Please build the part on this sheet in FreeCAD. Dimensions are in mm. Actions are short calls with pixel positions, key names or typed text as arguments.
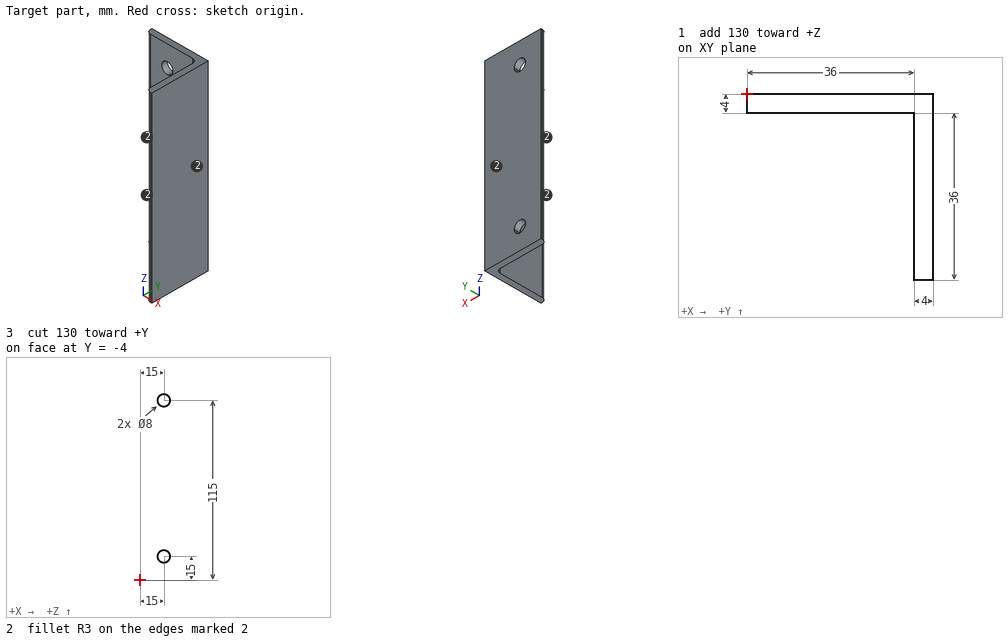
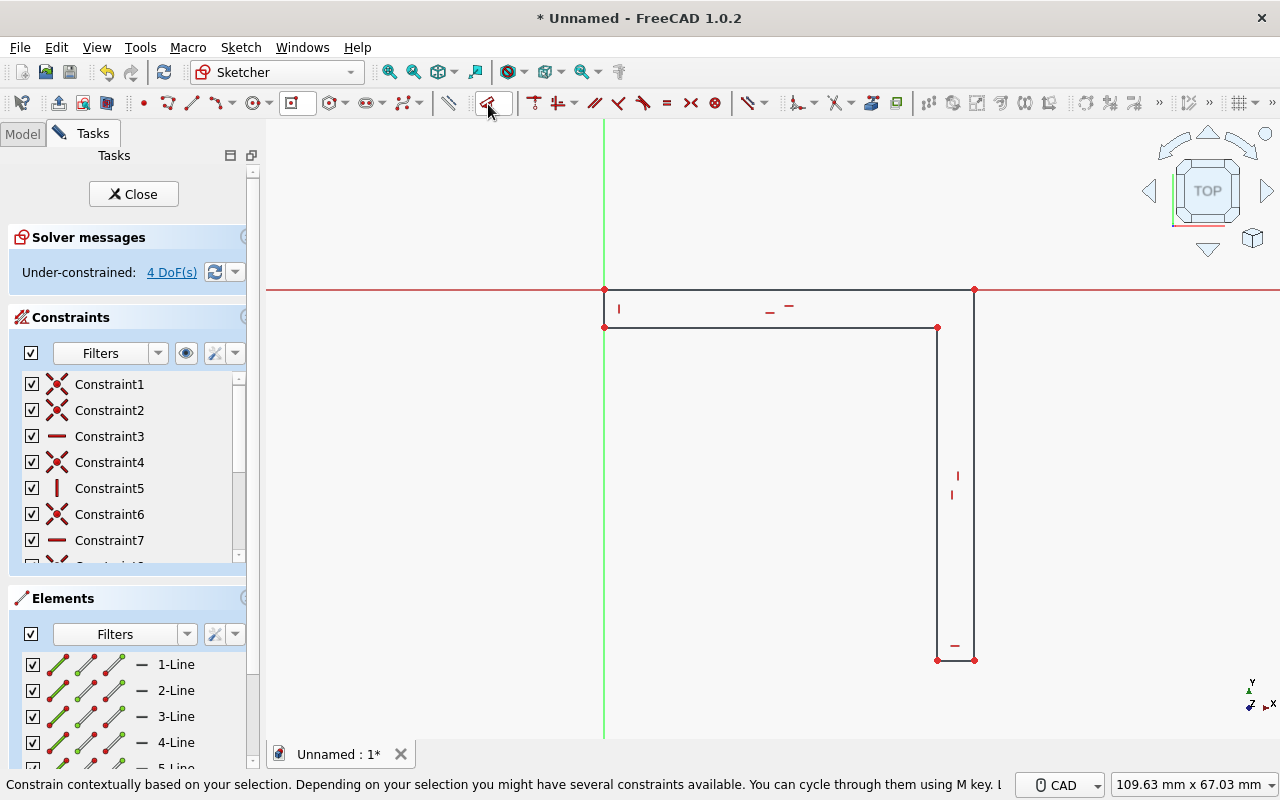
click(604, 301)
click(570, 309)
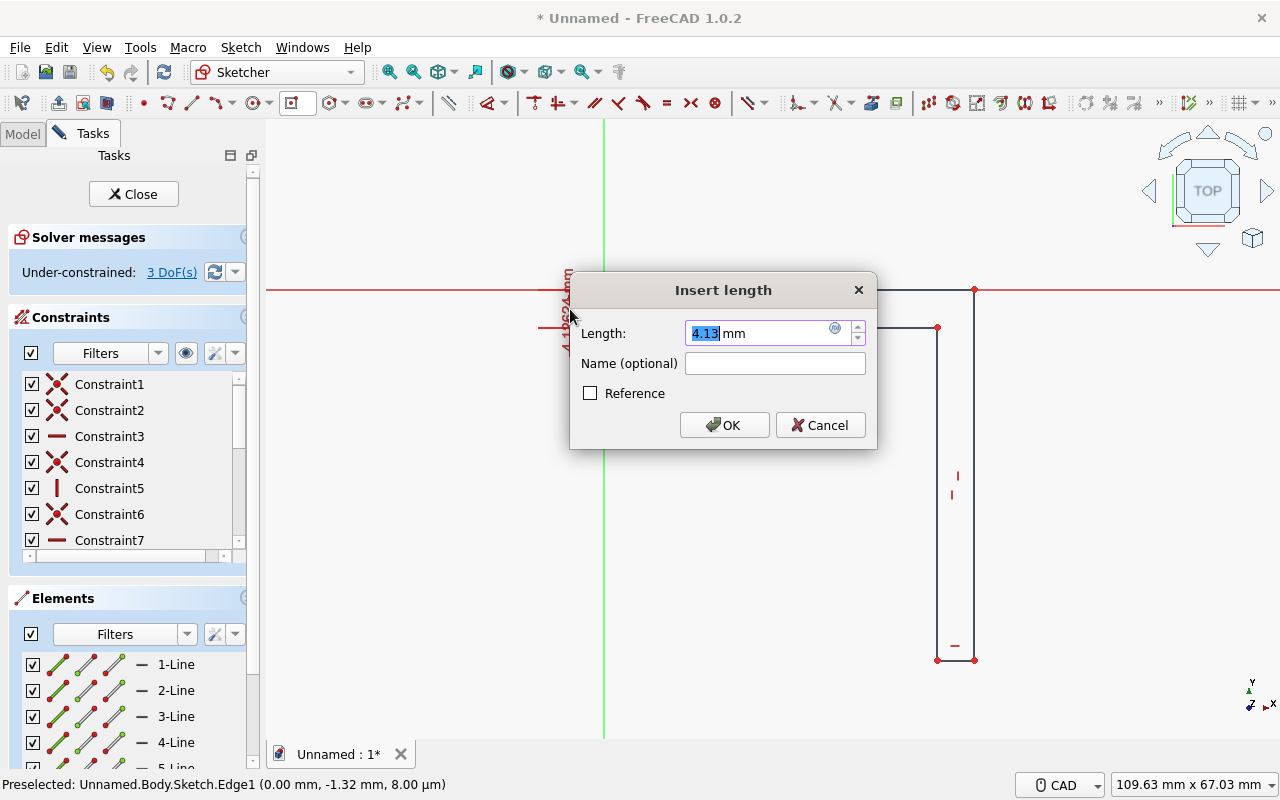
text(4)
key(Return)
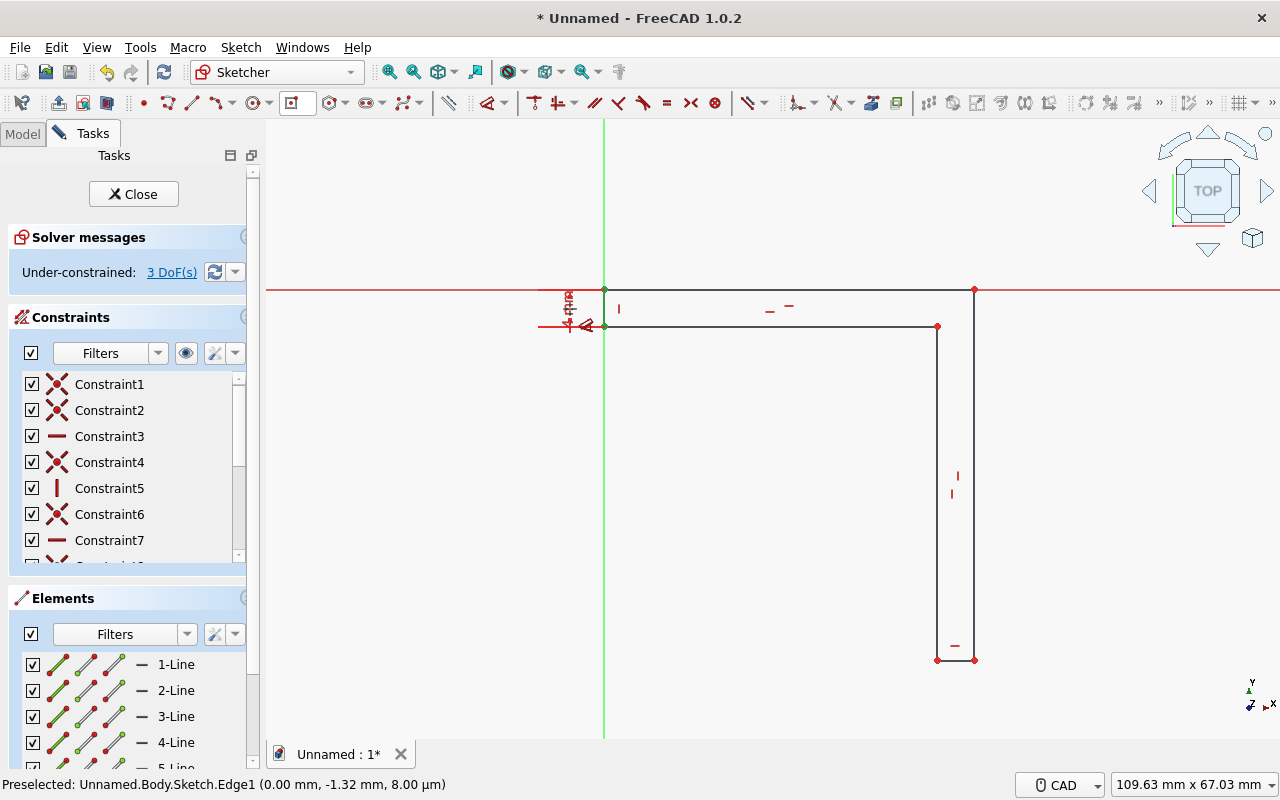
scroll(948, 661, up, 2)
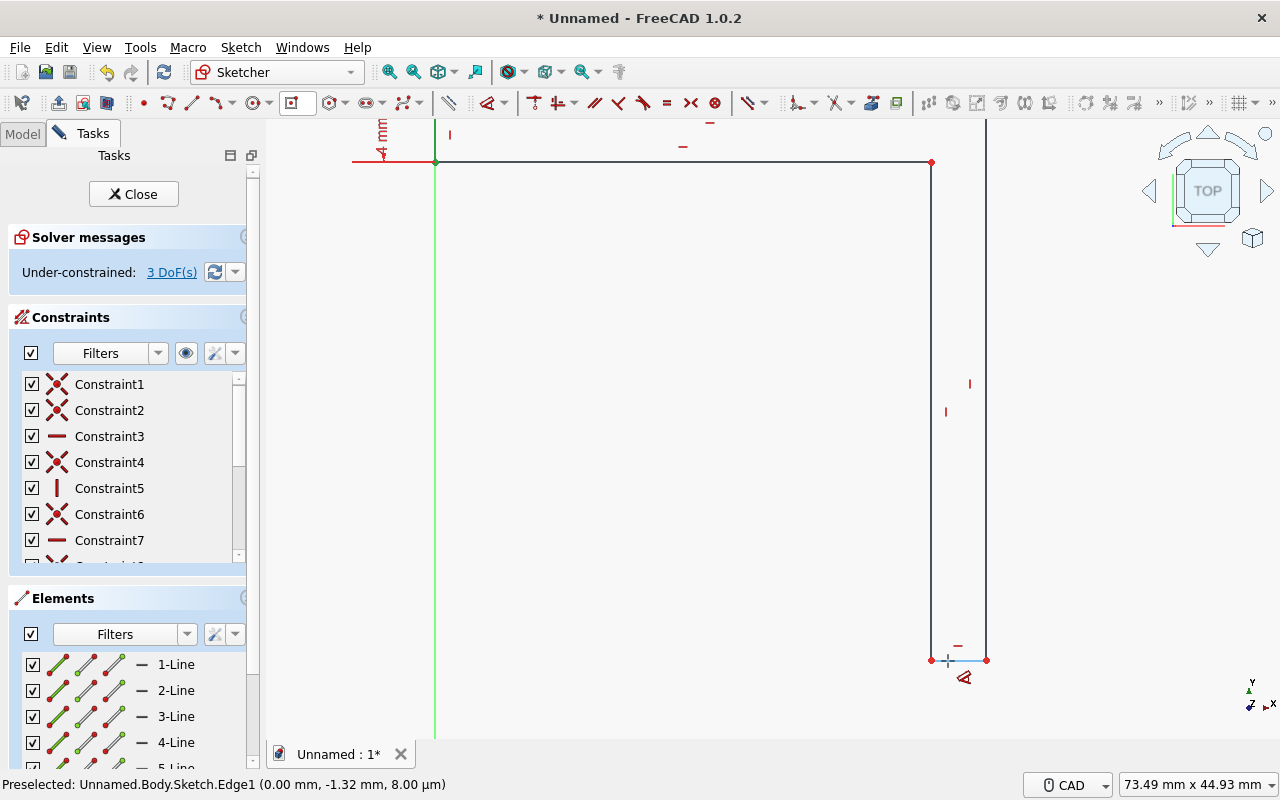
click(948, 661)
click(959, 695)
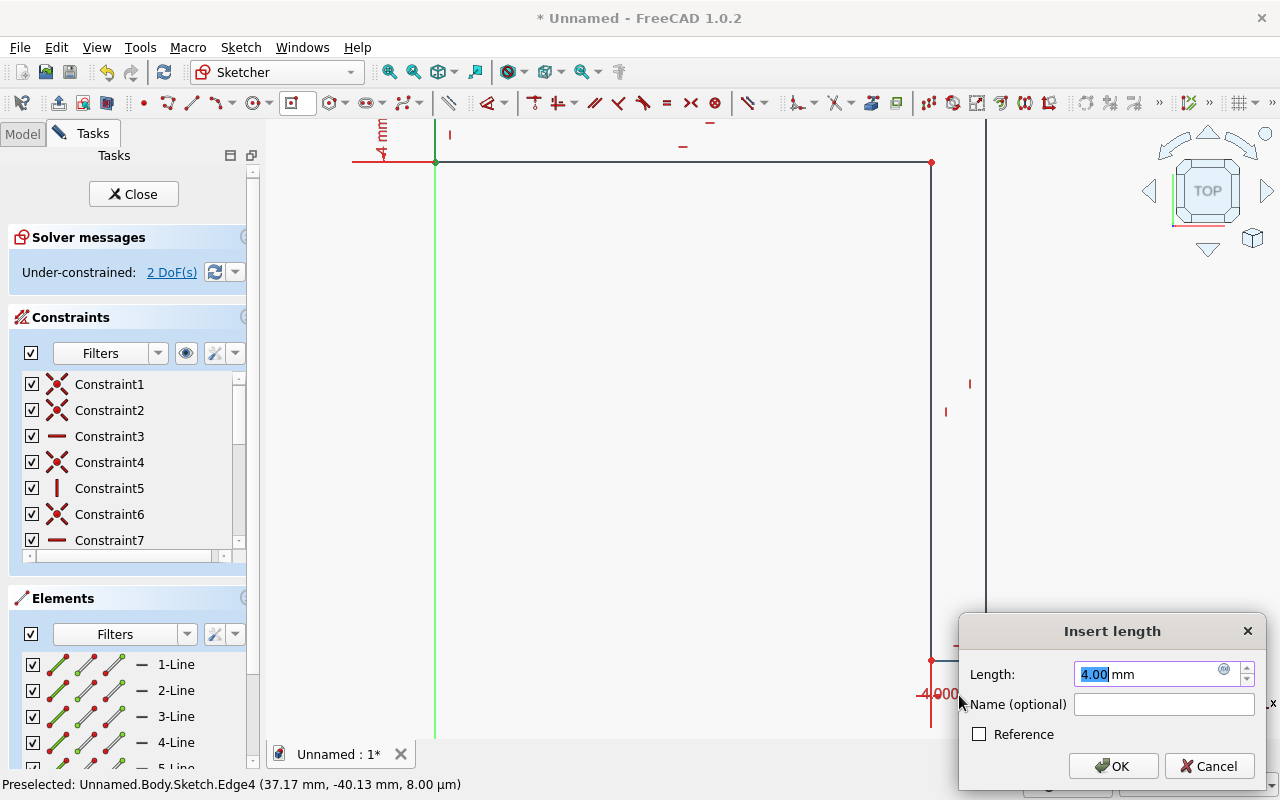
text(4)
key(Return)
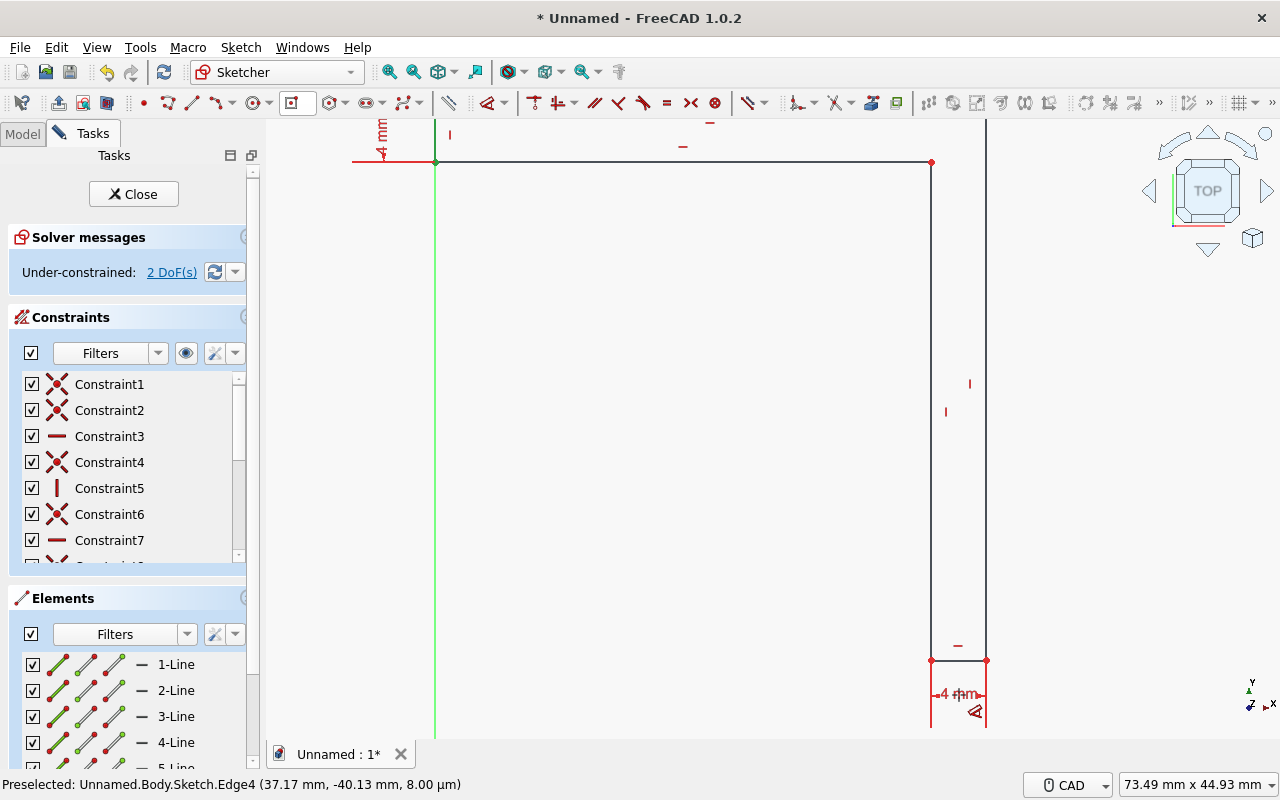
click(584, 162)
click(683, 196)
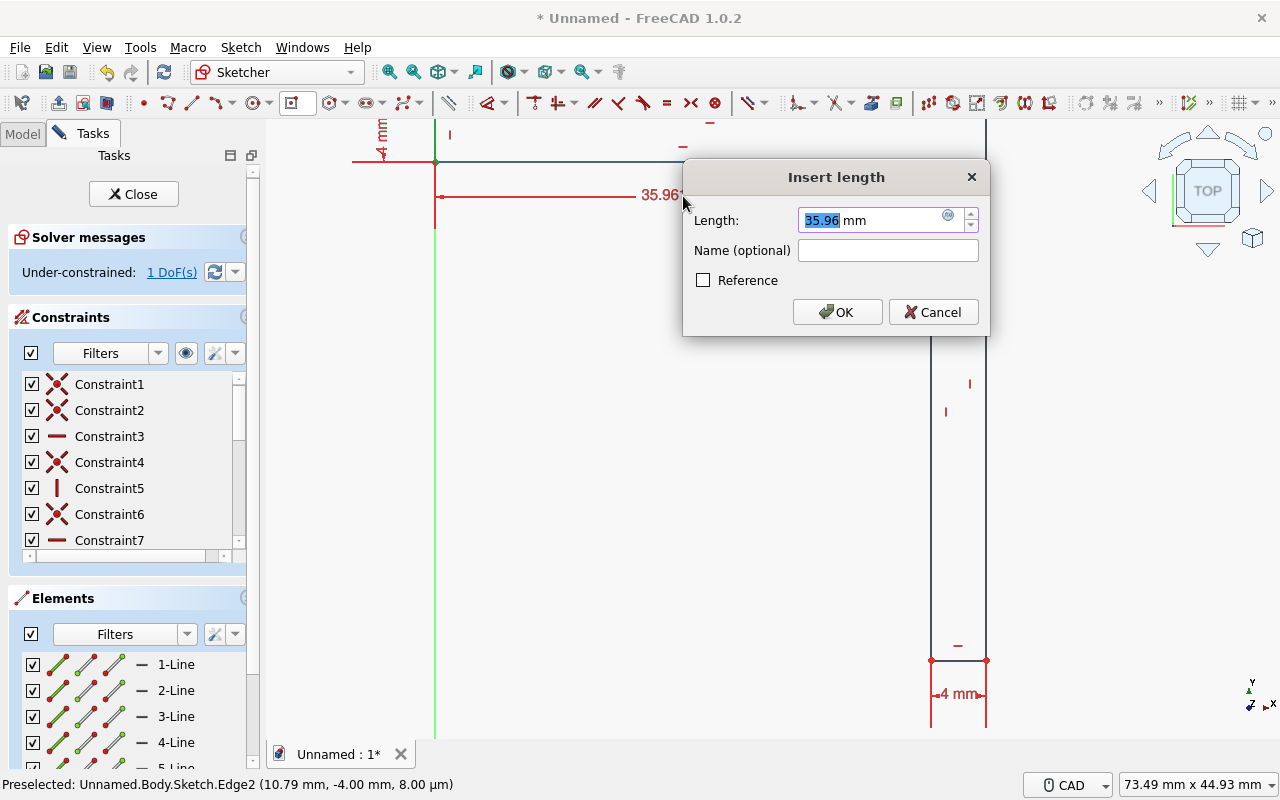
text(36)
key(Return)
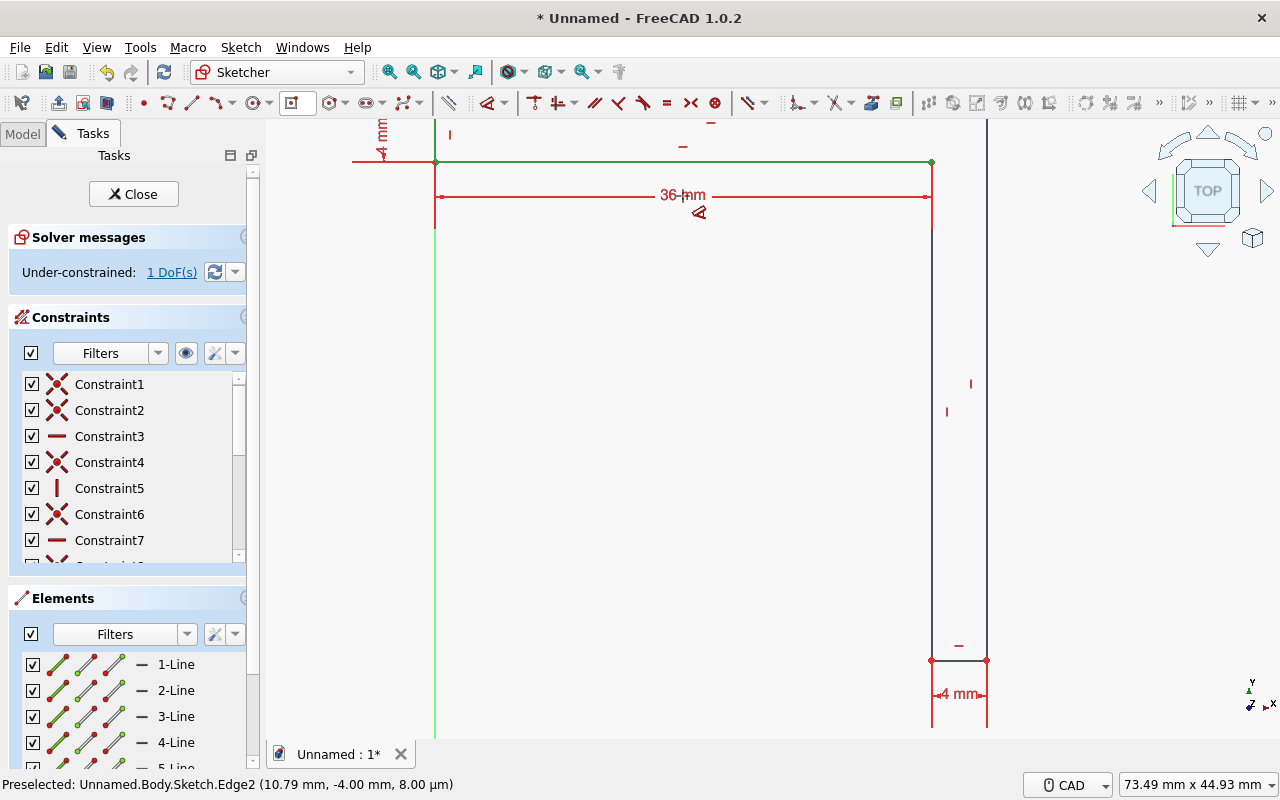
click(932, 312)
click(966, 411)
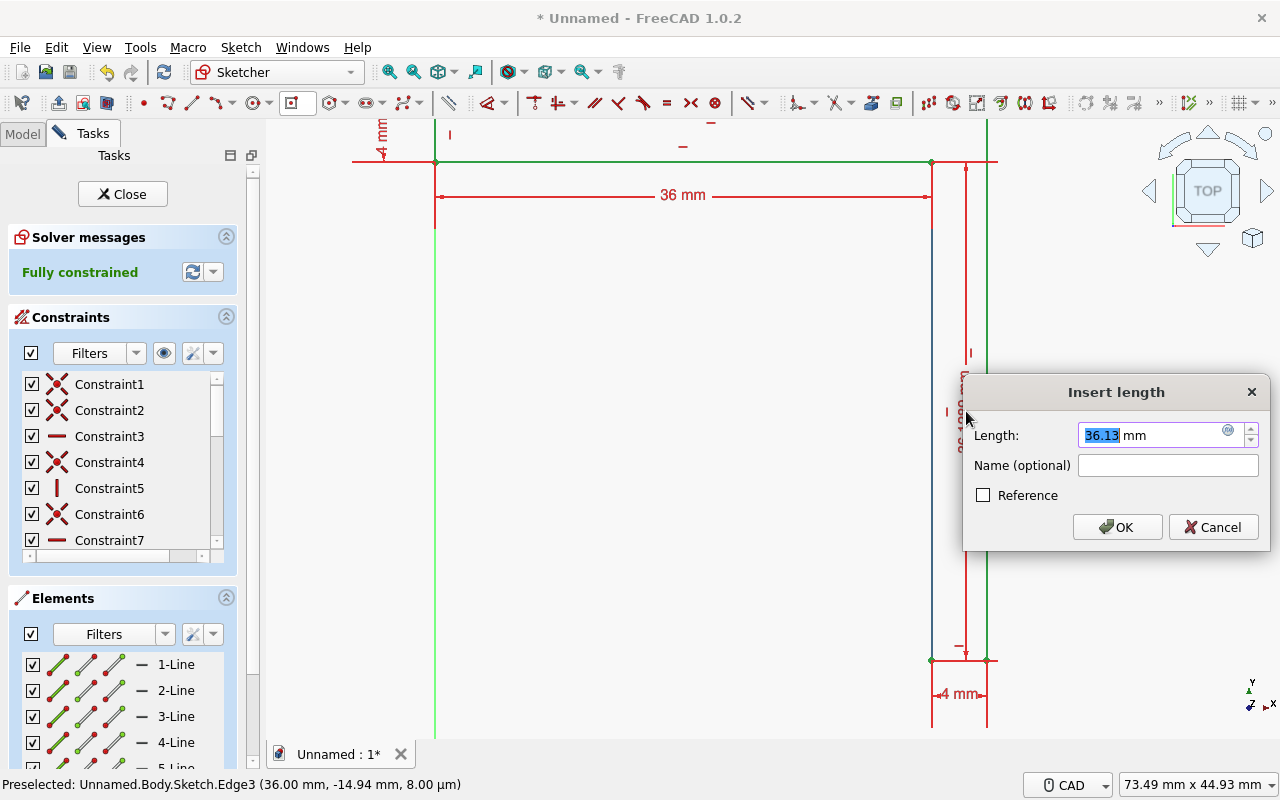
text(36)
key(Return)
key(Escape)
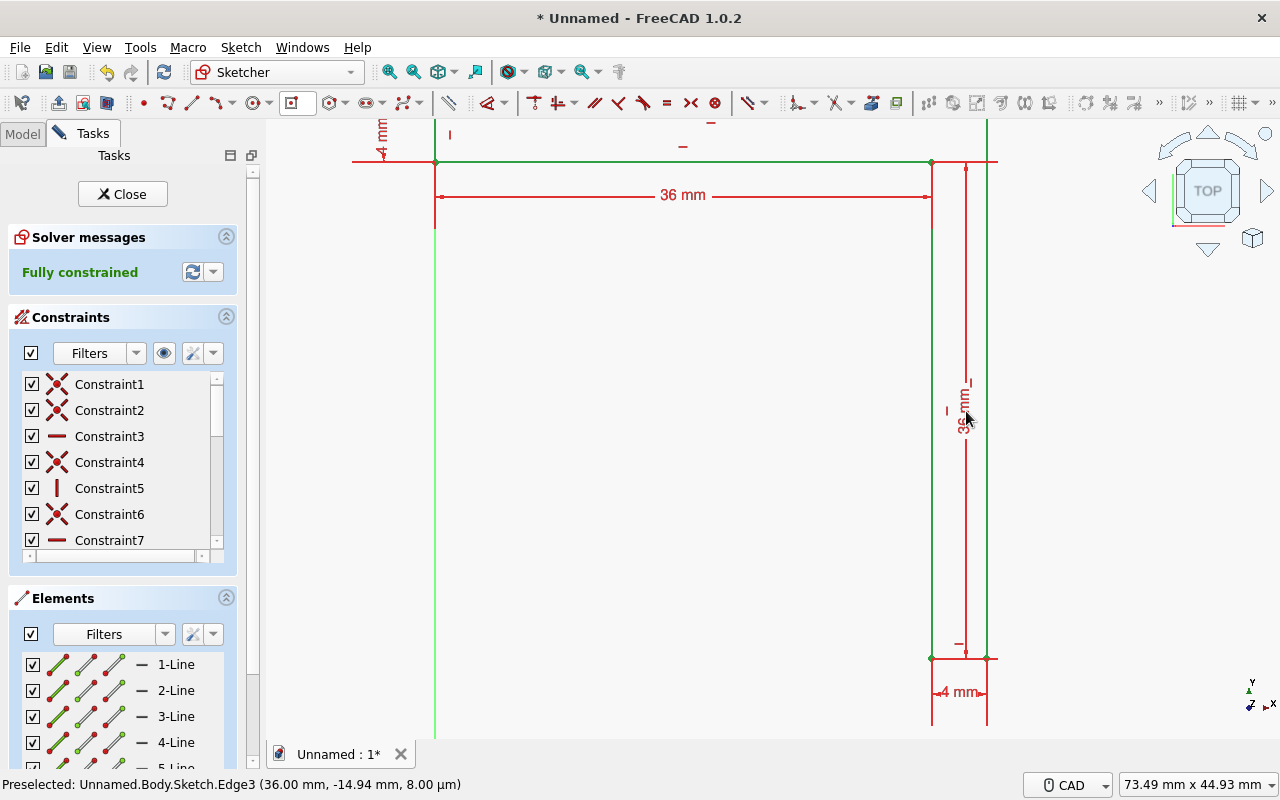
click(123, 194)